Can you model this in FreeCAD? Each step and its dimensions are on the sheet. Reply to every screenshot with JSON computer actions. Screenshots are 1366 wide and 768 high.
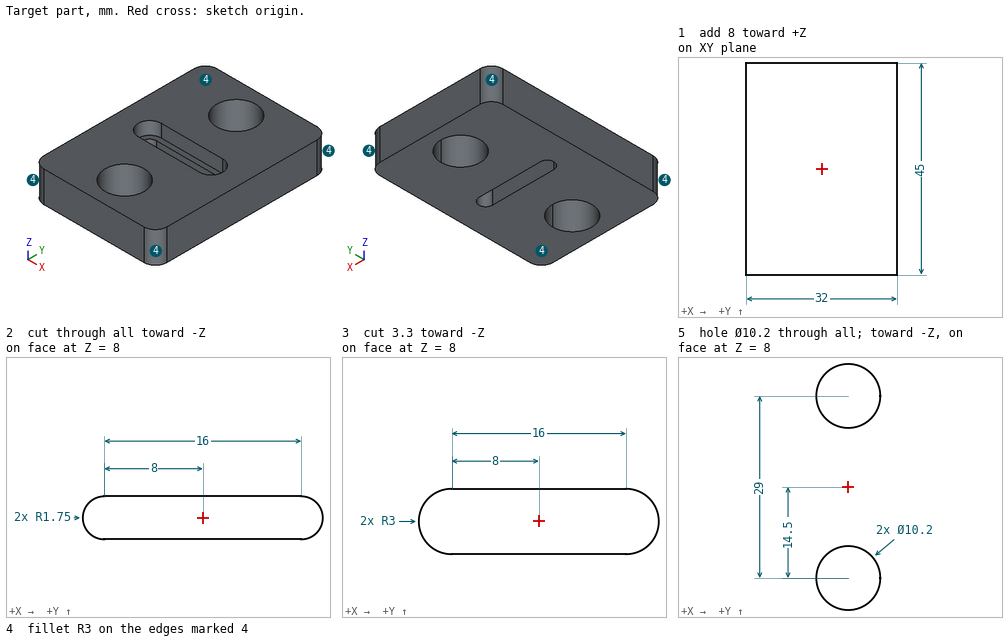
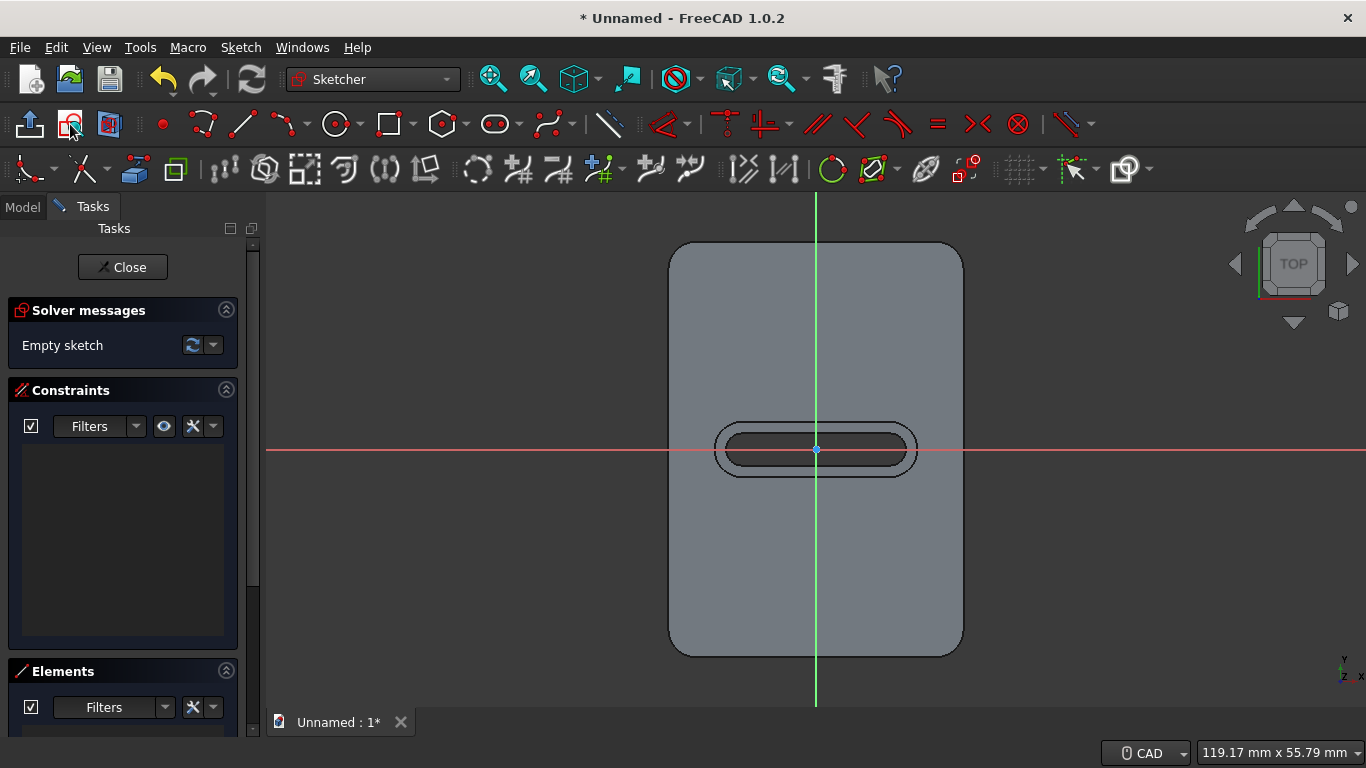
{"action": "left_click", "coordinate": [336, 124]}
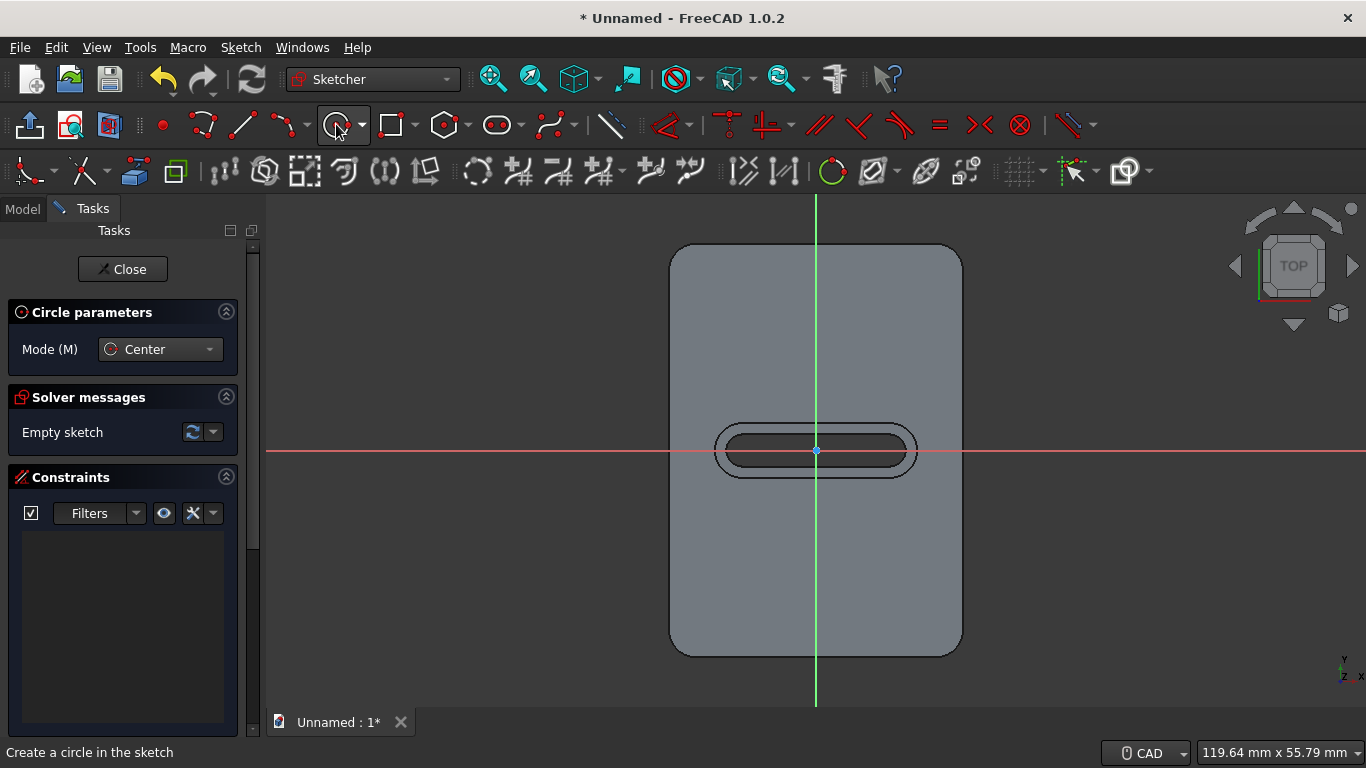
{"action": "left_click", "coordinate": [816, 584]}
{"action": "mouse_move", "coordinate": [849, 551]}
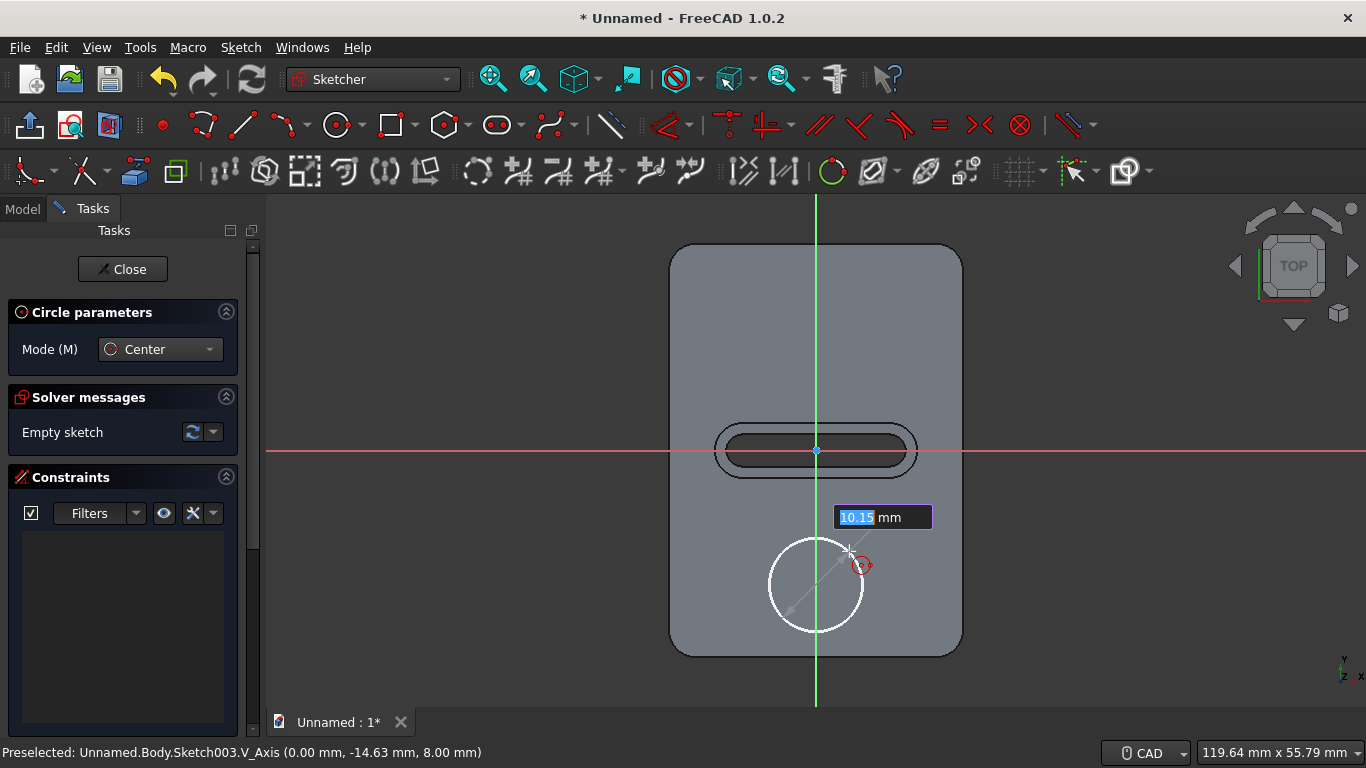
{"action": "type", "text": "10.2"}
{"action": "key", "text": "Return"}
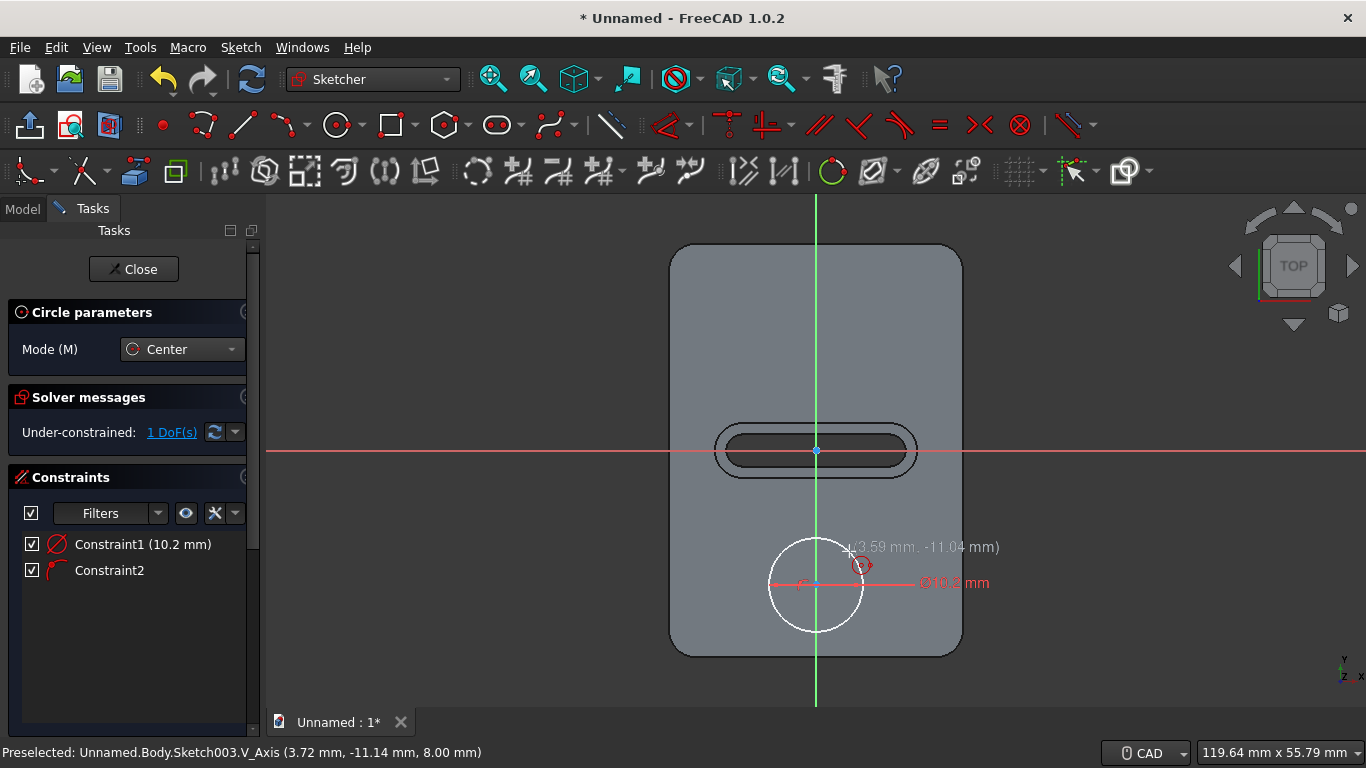
{"action": "left_click", "coordinate": [816, 317]}
{"action": "mouse_move", "coordinate": [849, 284]}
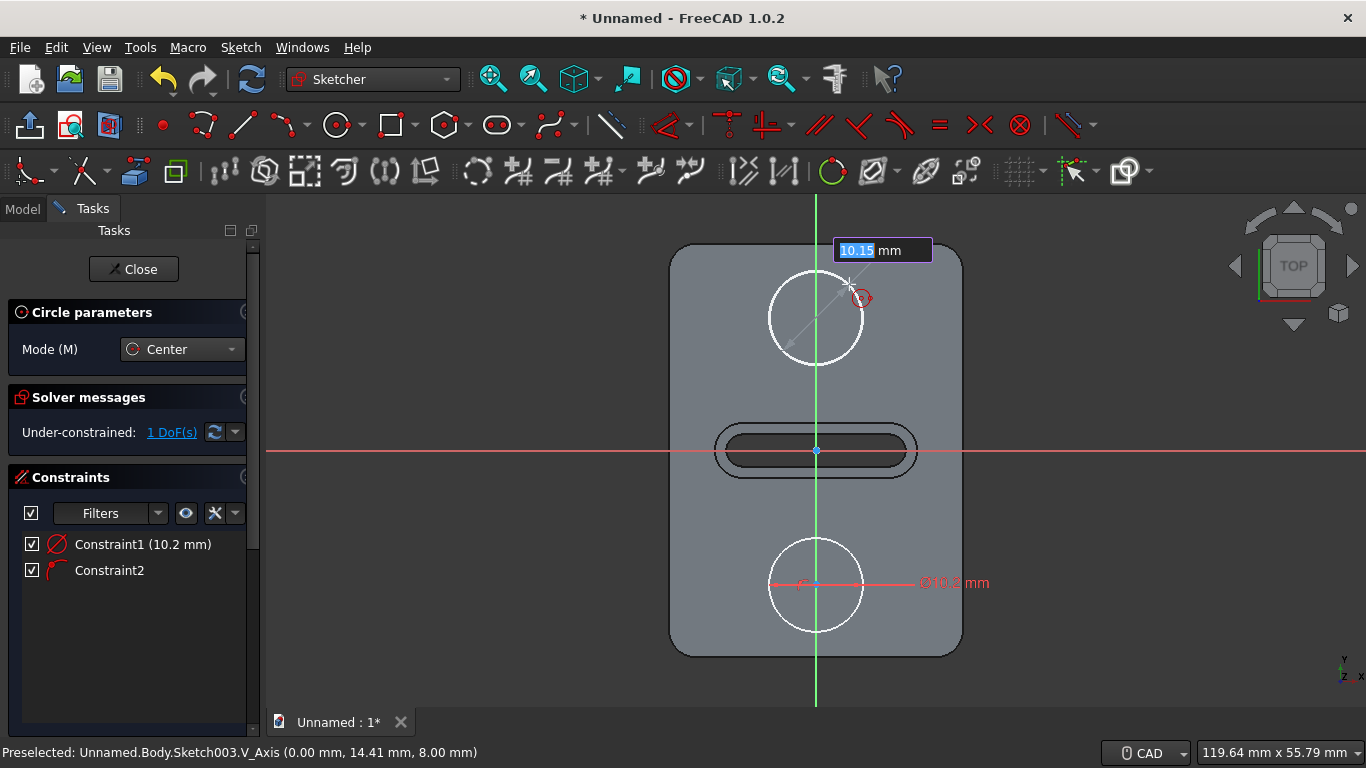
{"action": "type", "text": "10.2"}
{"action": "key", "text": "Return"}
{"action": "key", "text": "Escape"}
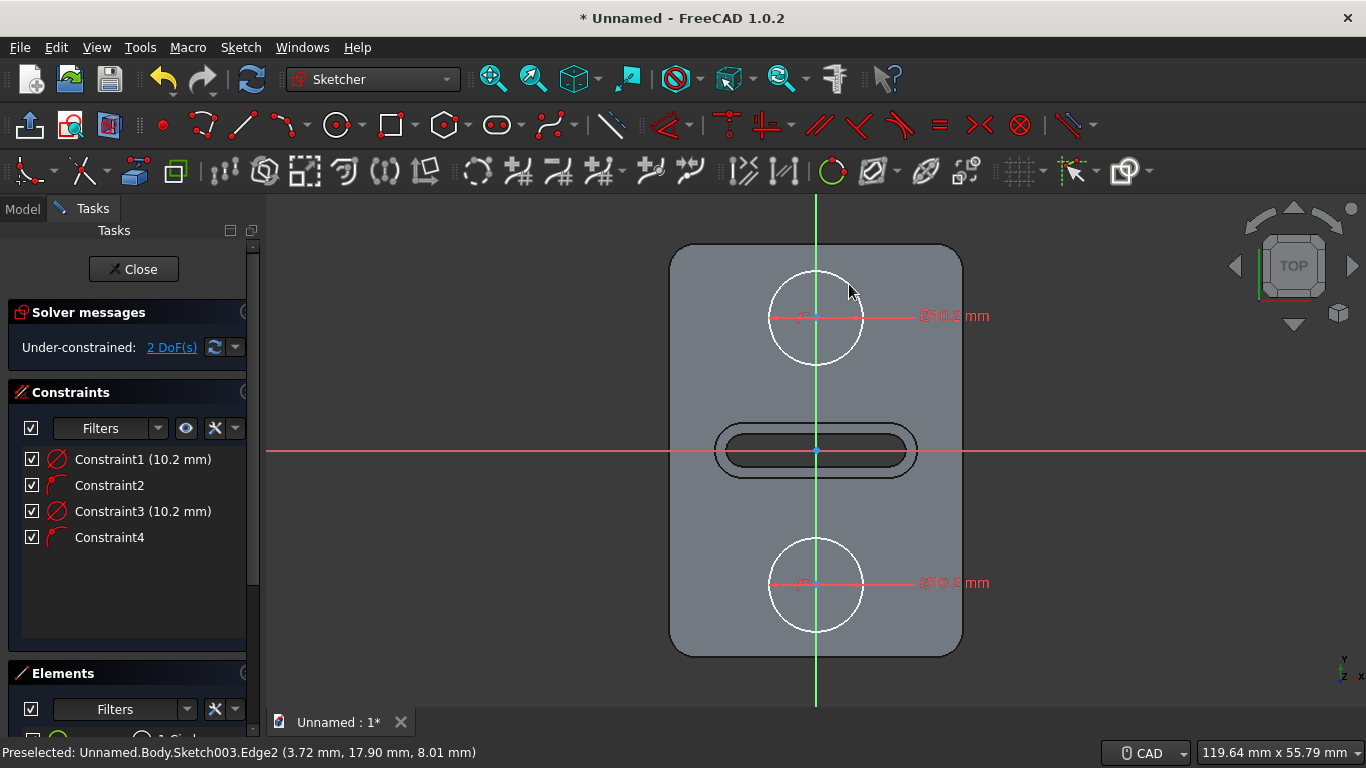
{"action": "left_click", "coordinate": [666, 126]}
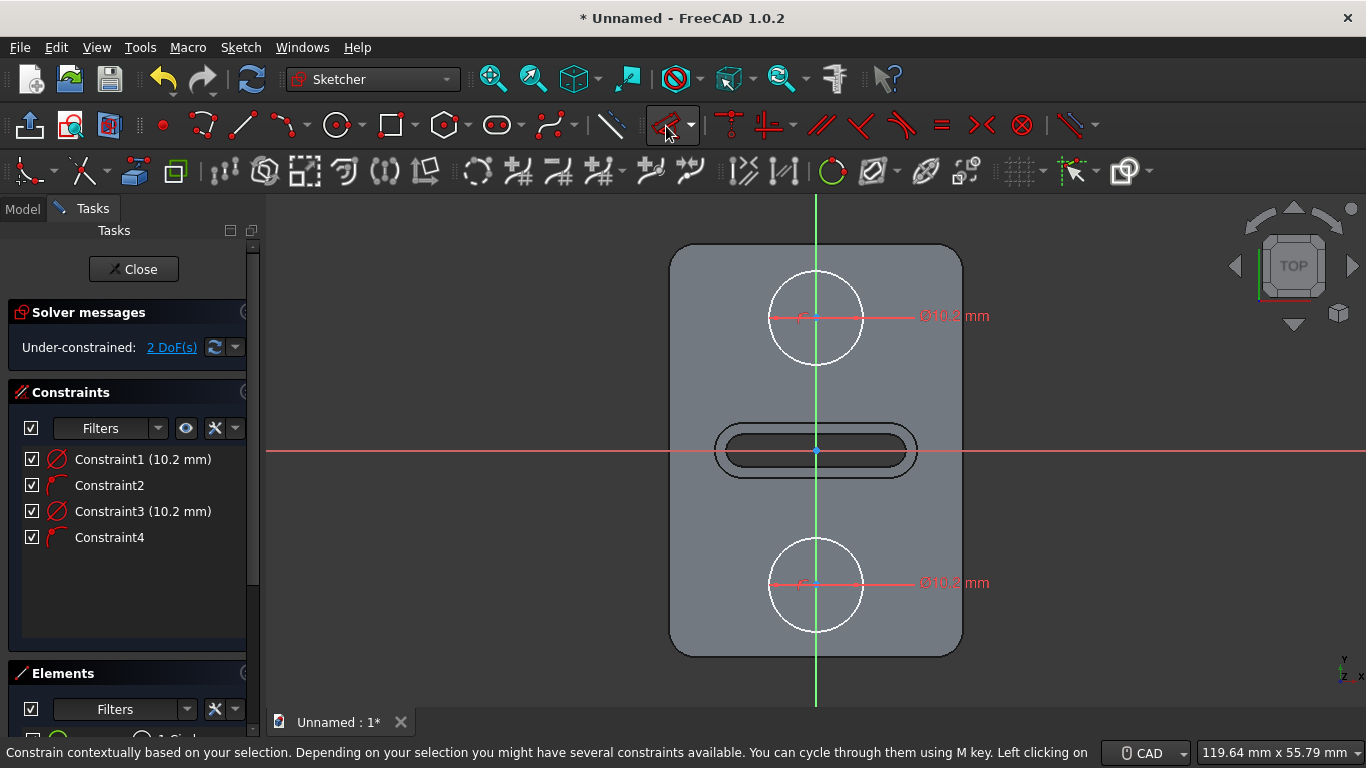
{"action": "left_click", "coordinate": [816, 585]}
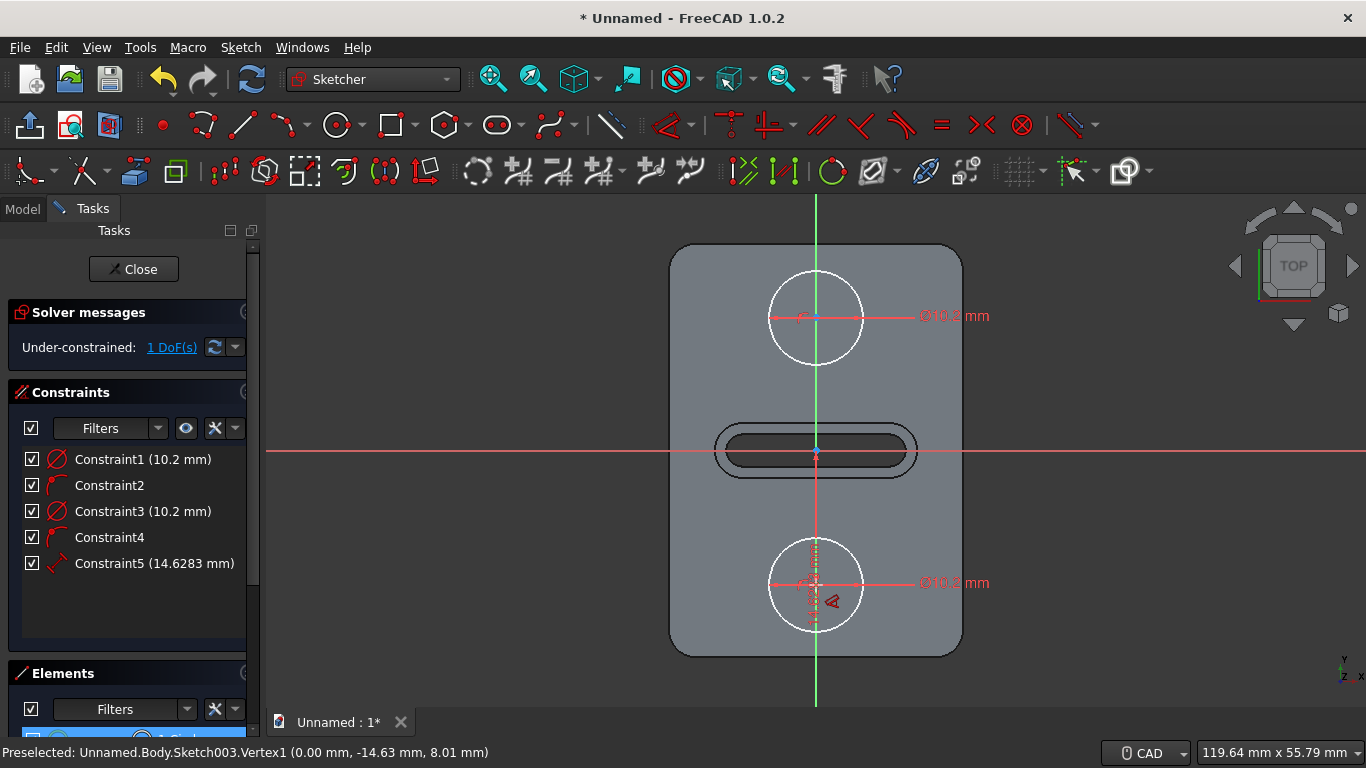
{"action": "left_click", "coordinate": [816, 318]}
{"action": "left_click", "coordinate": [850, 390]}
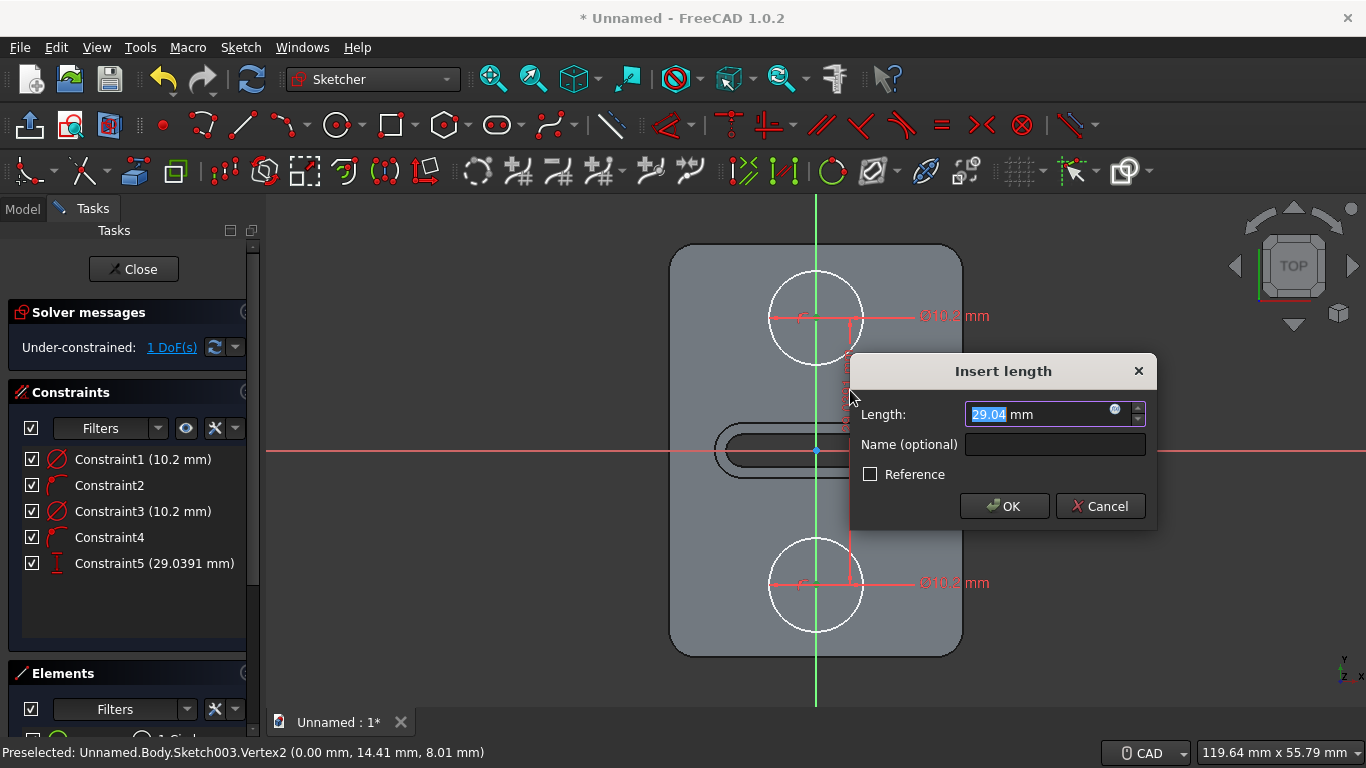
{"action": "type", "text": "29"}
{"action": "key", "text": "Return"}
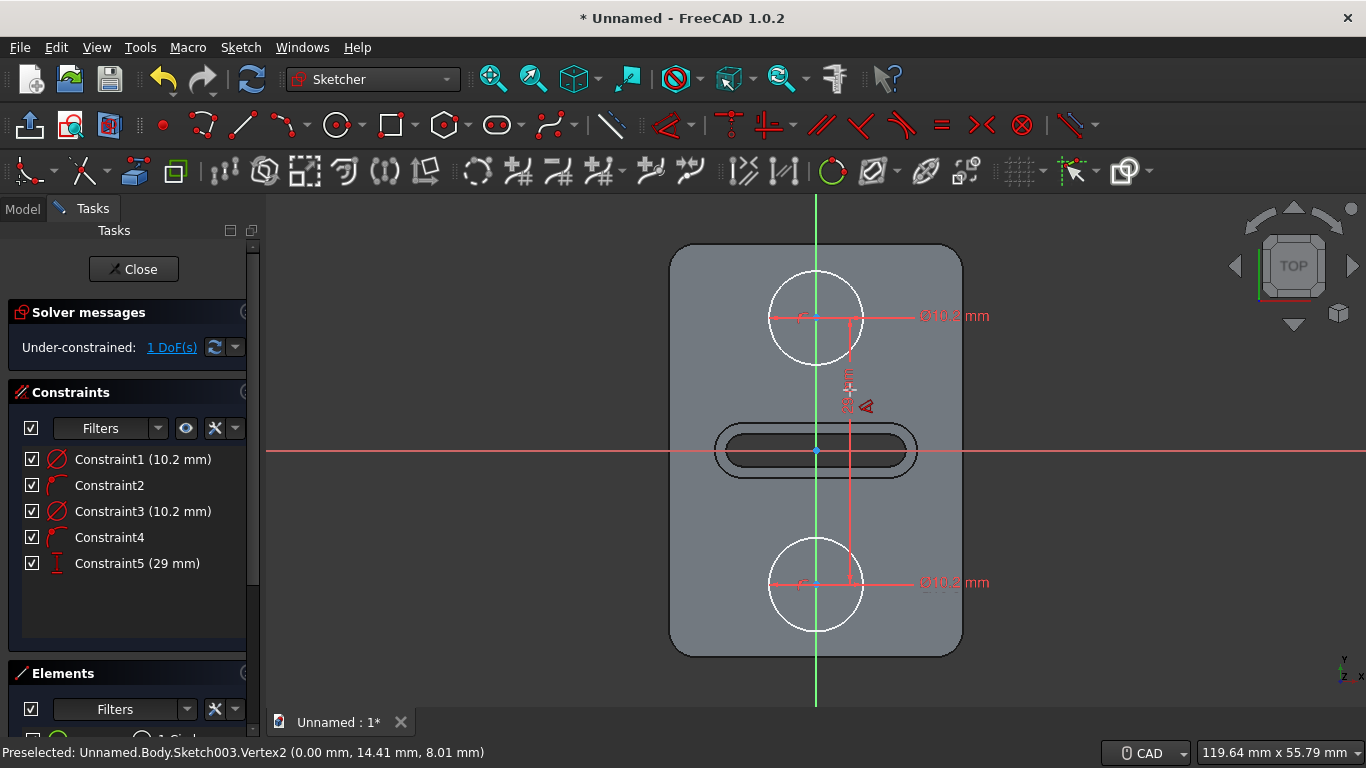
{"action": "left_click", "coordinate": [816, 585]}
{"action": "left_click", "coordinate": [850, 518]}